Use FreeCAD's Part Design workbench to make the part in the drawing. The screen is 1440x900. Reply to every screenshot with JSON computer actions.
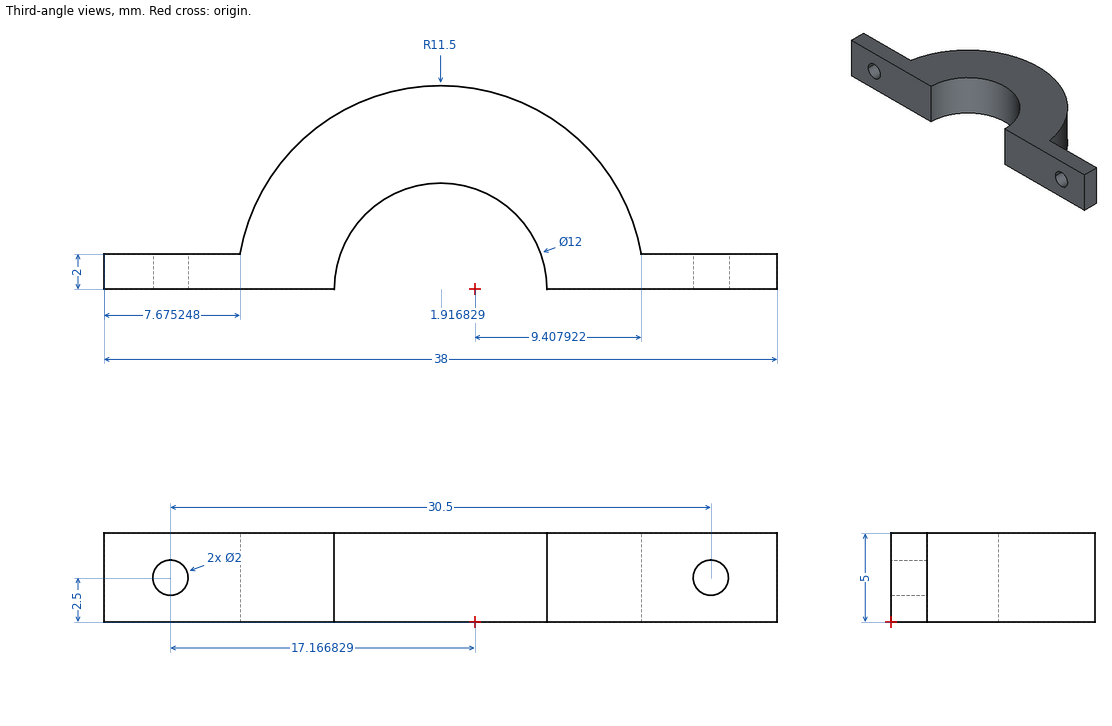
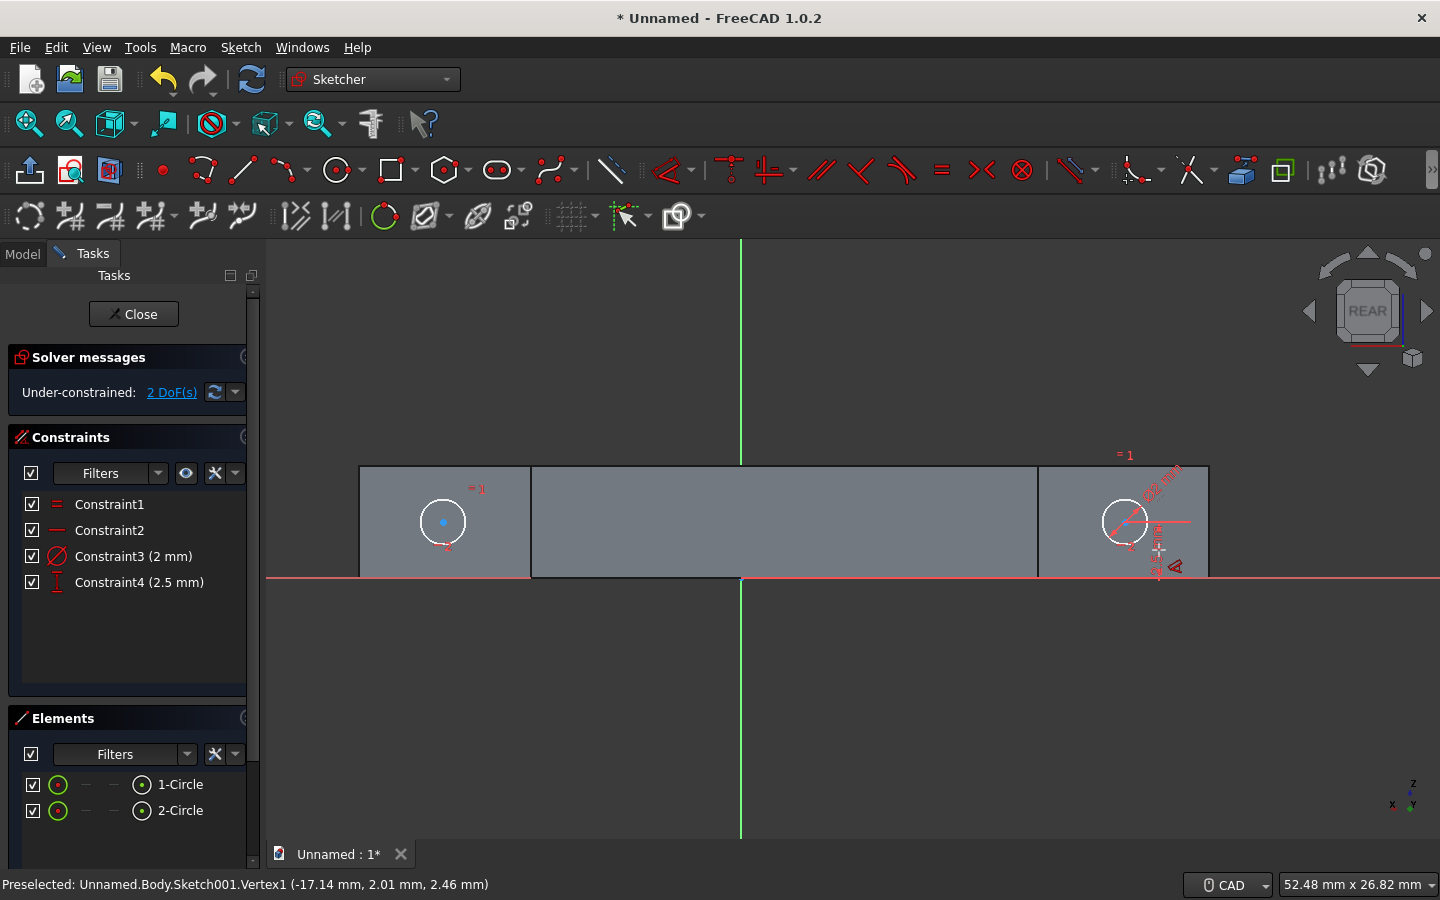
{"action": "left_click", "coordinate": [1125, 522]}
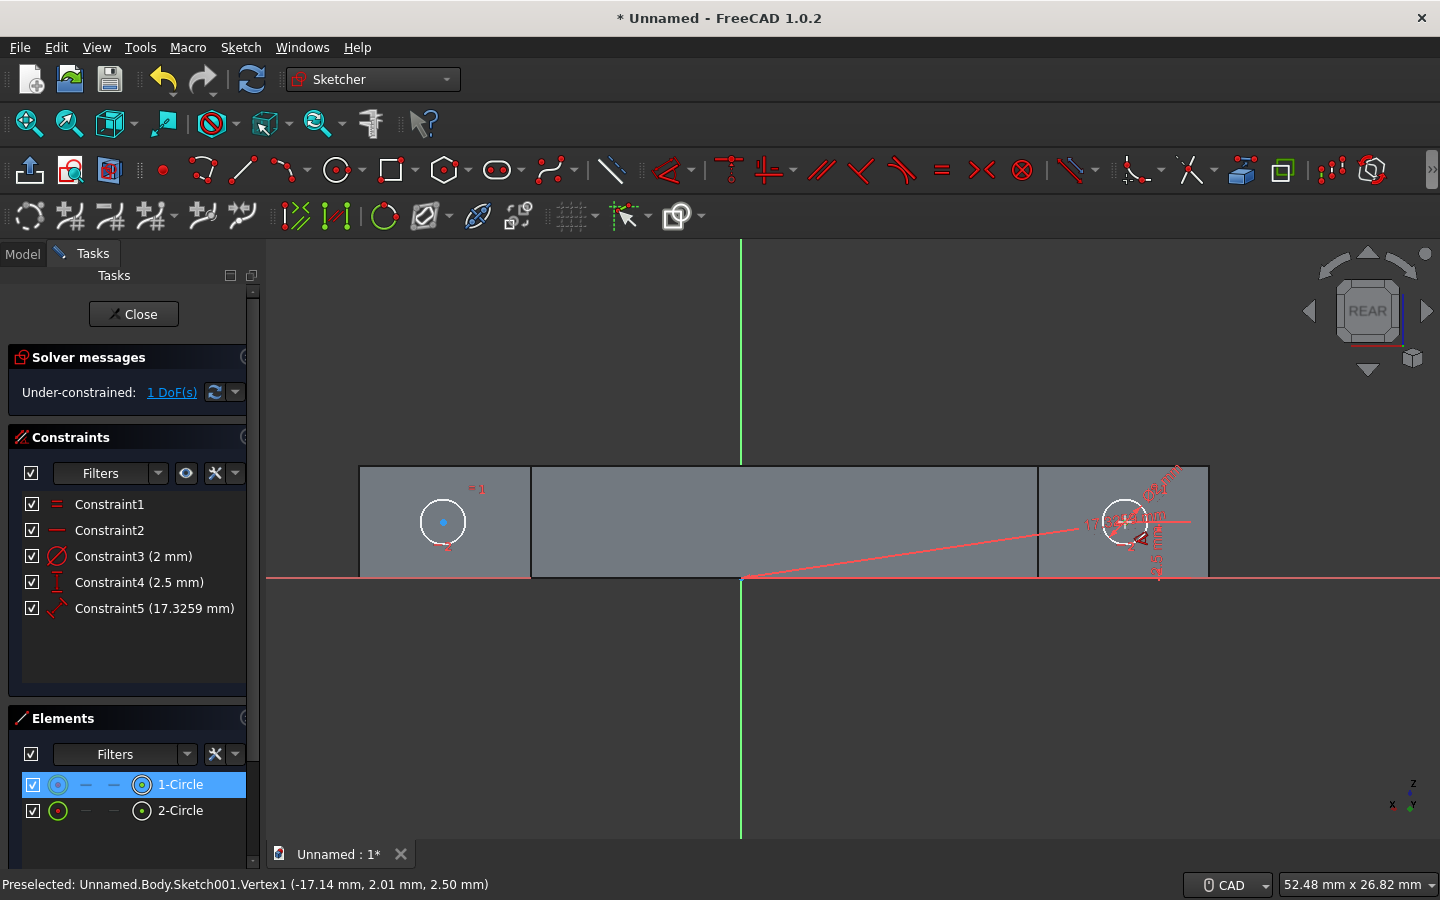
{"action": "left_click", "coordinate": [443, 522]}
{"action": "left_click", "coordinate": [784, 488]}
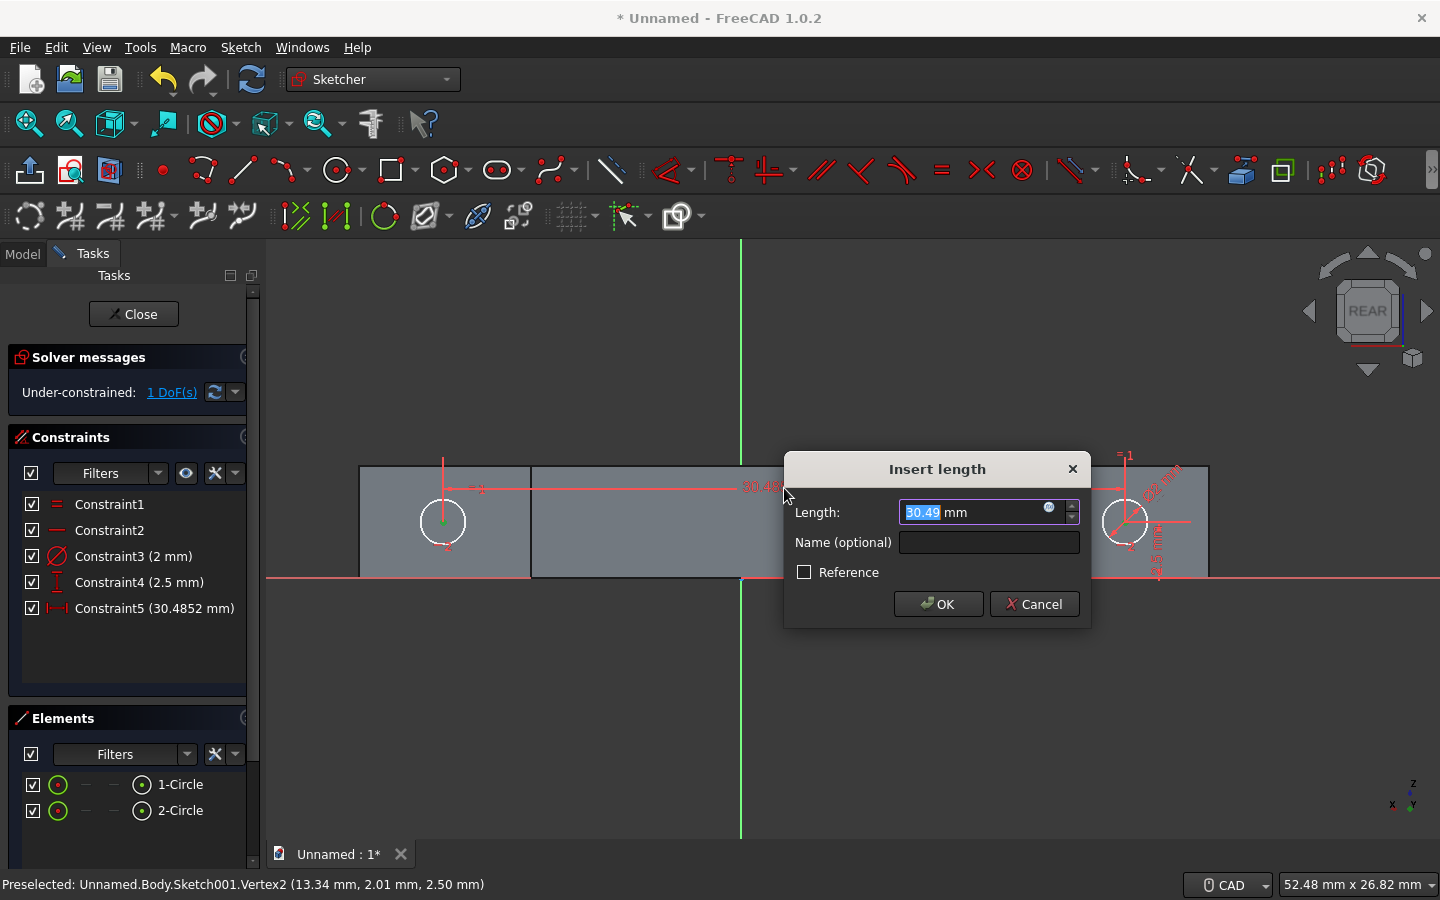
{"action": "type", "text": "30.5"}
{"action": "key", "text": "Return"}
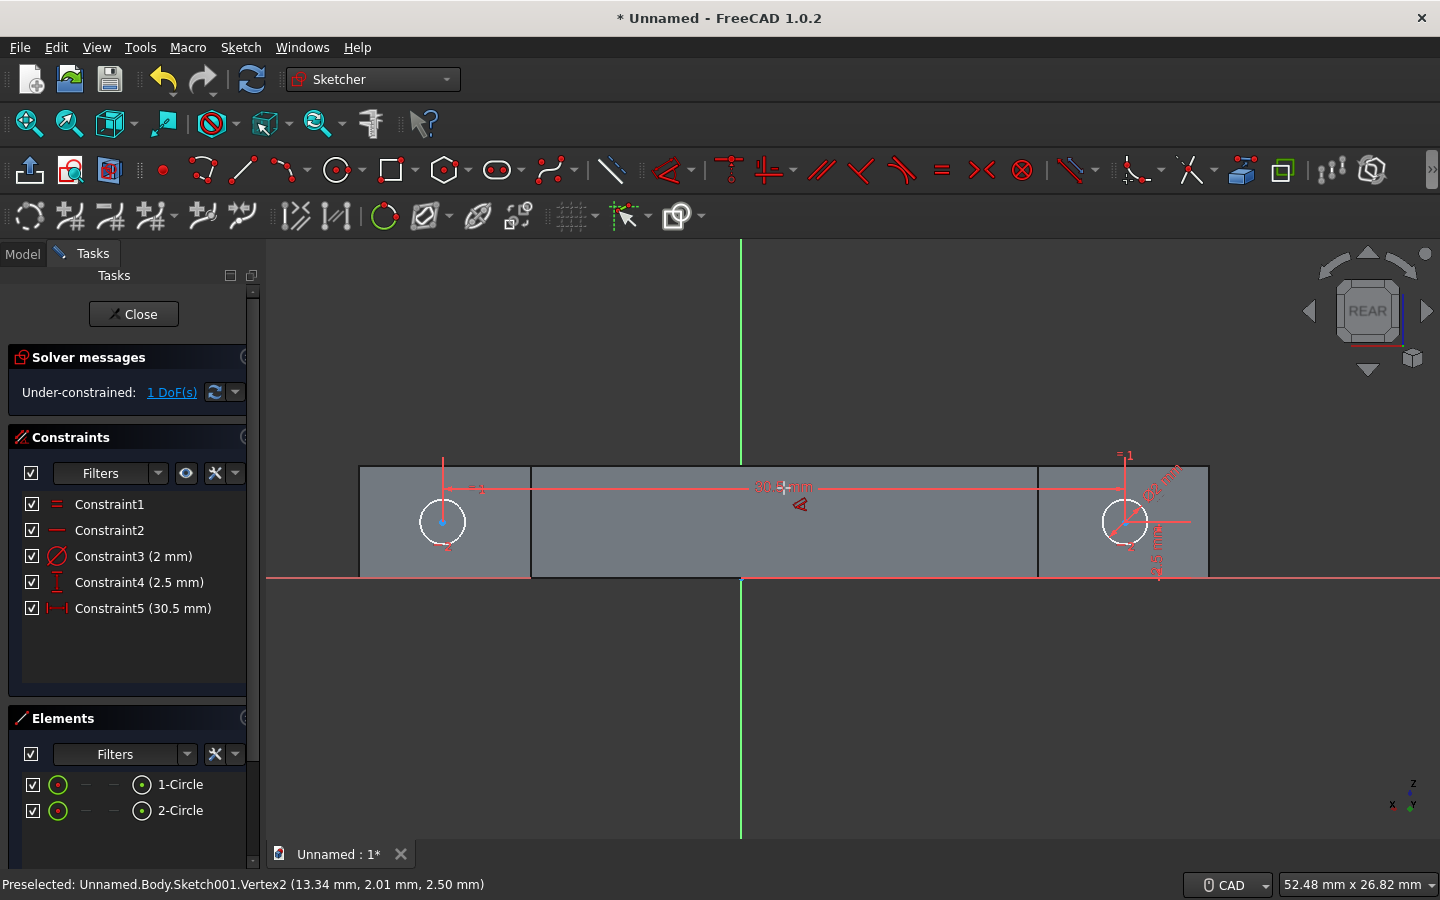
{"action": "left_click", "coordinate": [1125, 522]}
{"action": "left_click", "coordinate": [933, 612]}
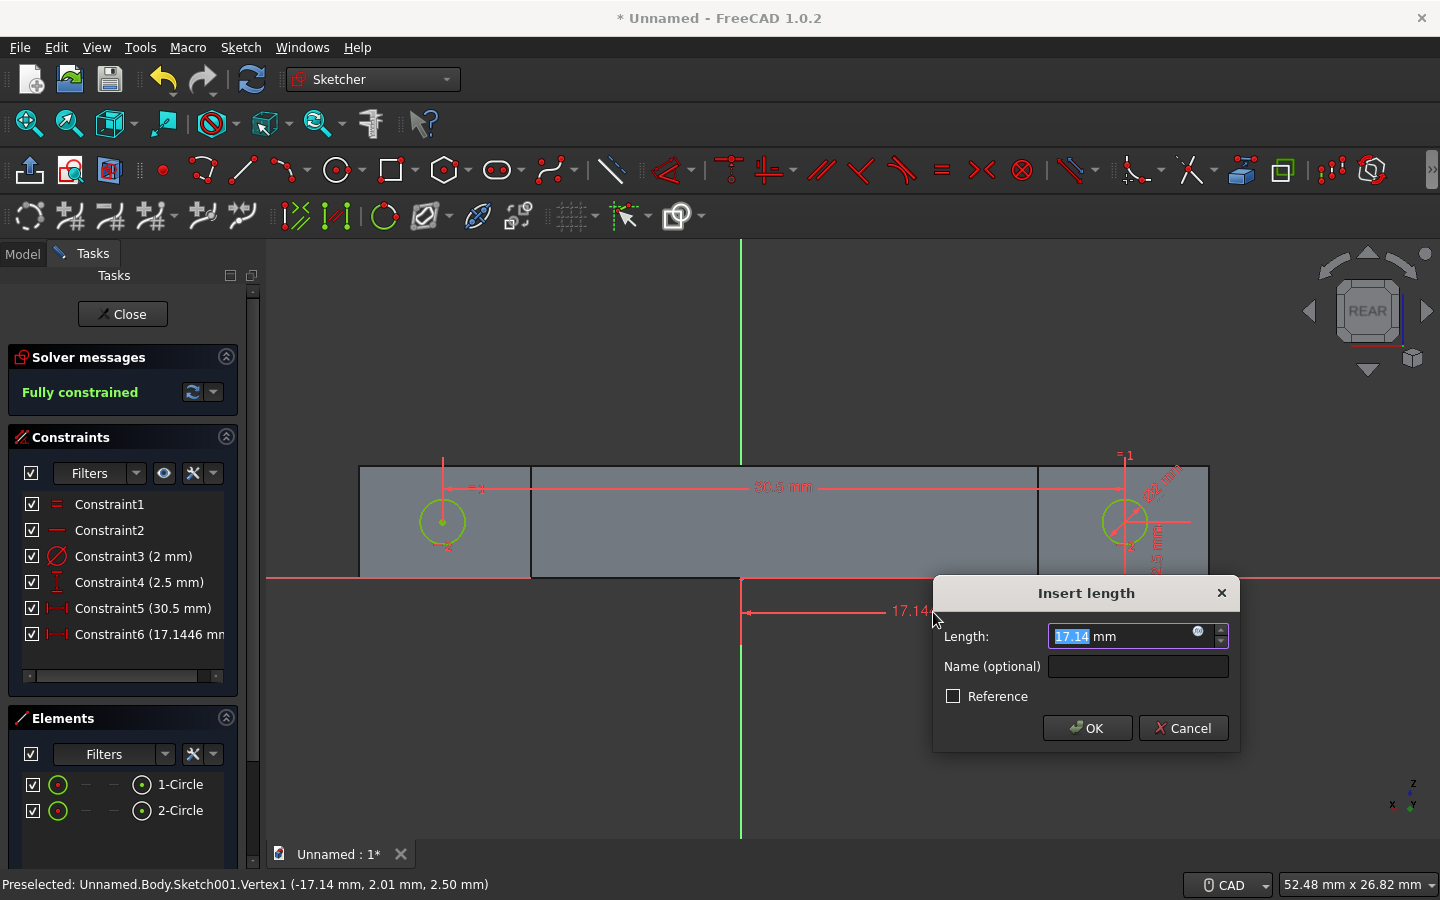
{"action": "type", "text": "17.166829"}
{"action": "key", "text": "Return"}
{"action": "key", "text": "Escape"}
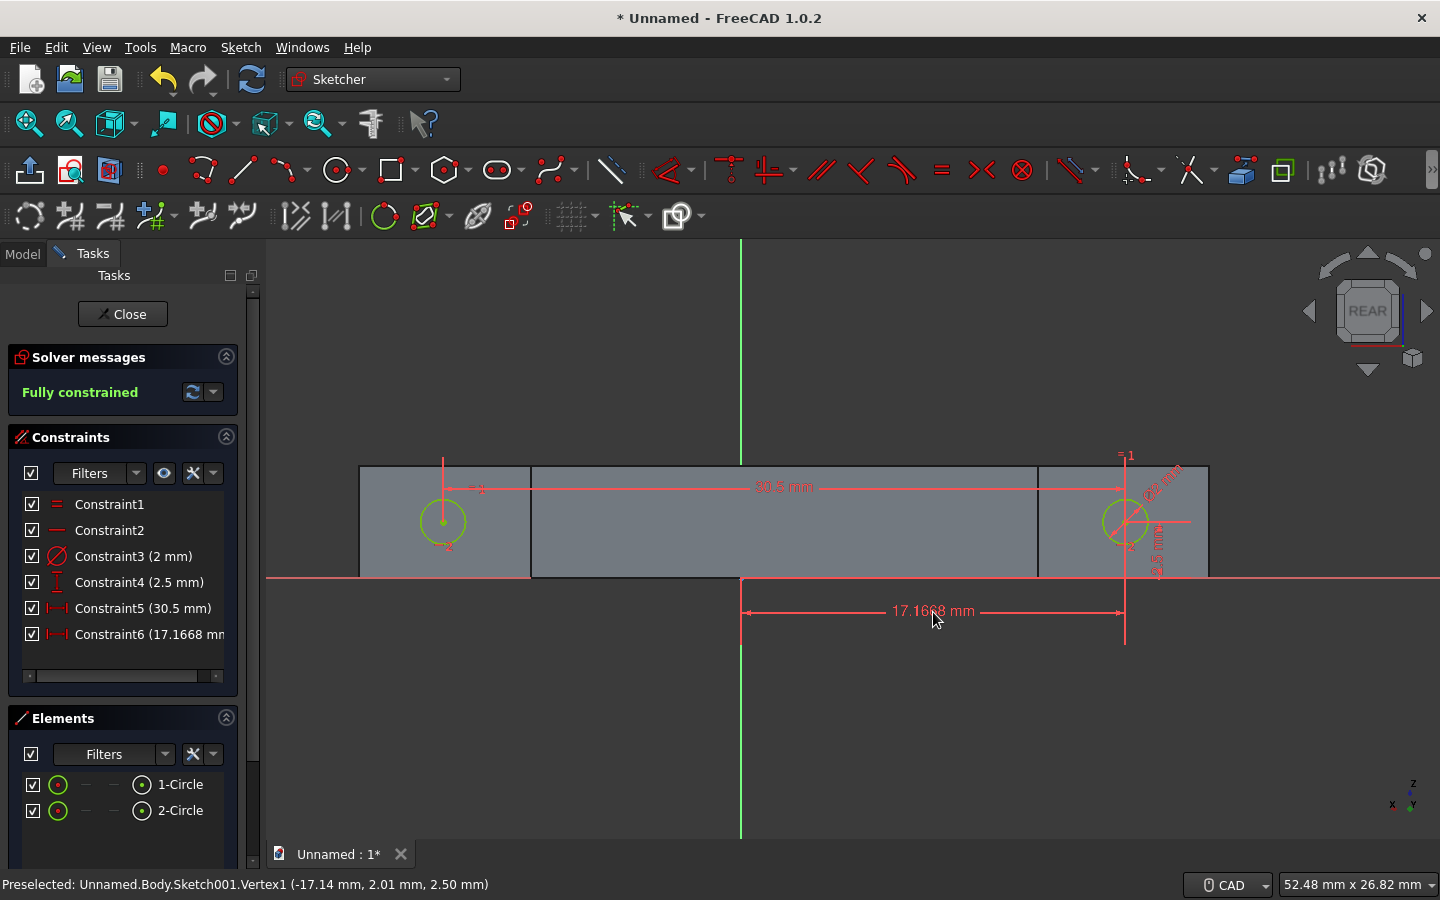
{"action": "left_click", "coordinate": [123, 314]}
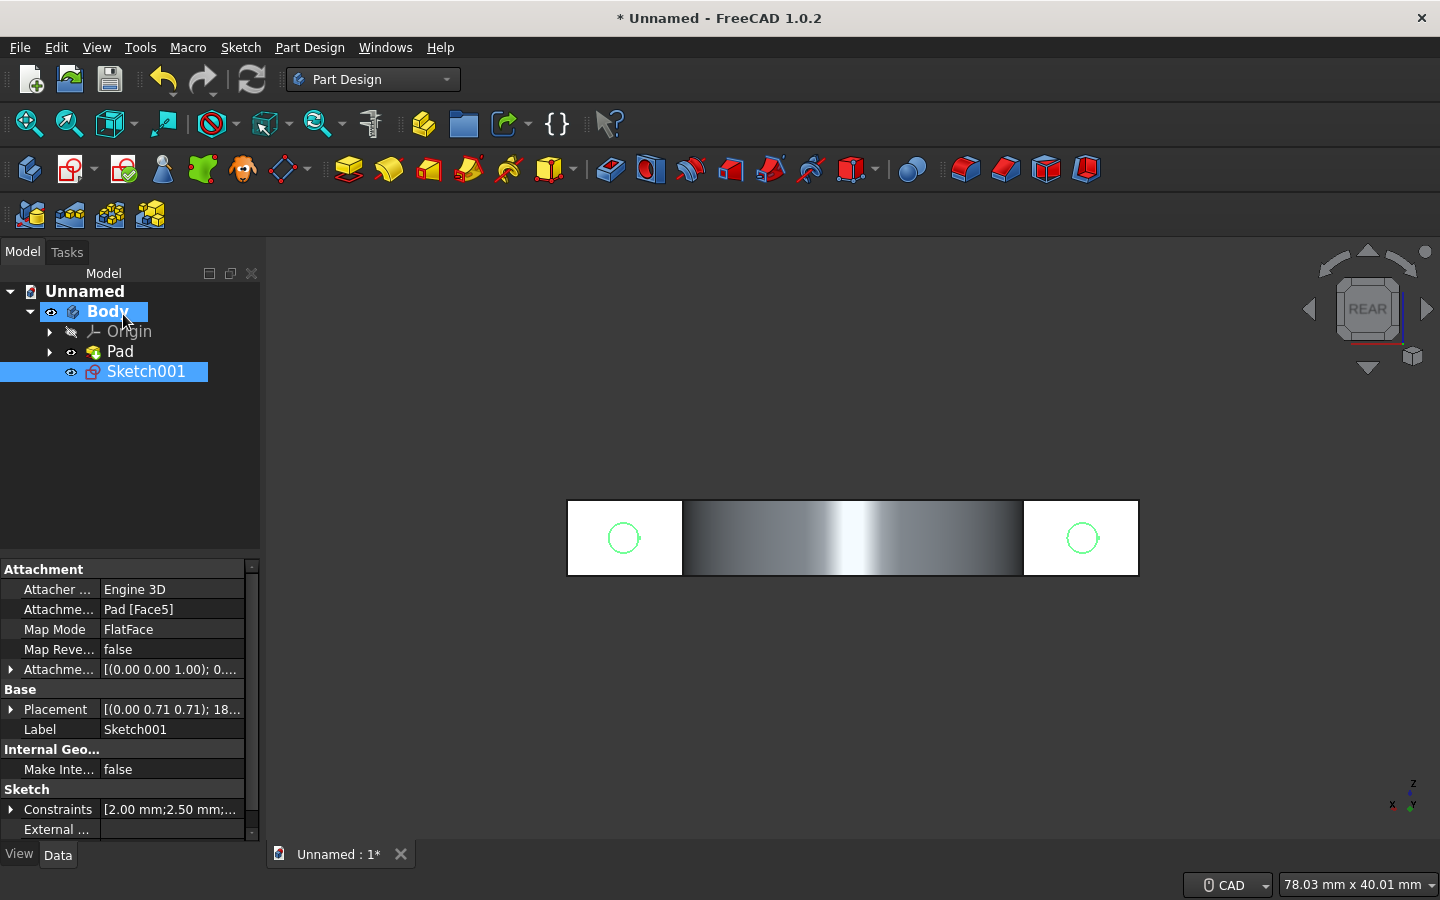
{"action": "left_click", "coordinate": [612, 170]}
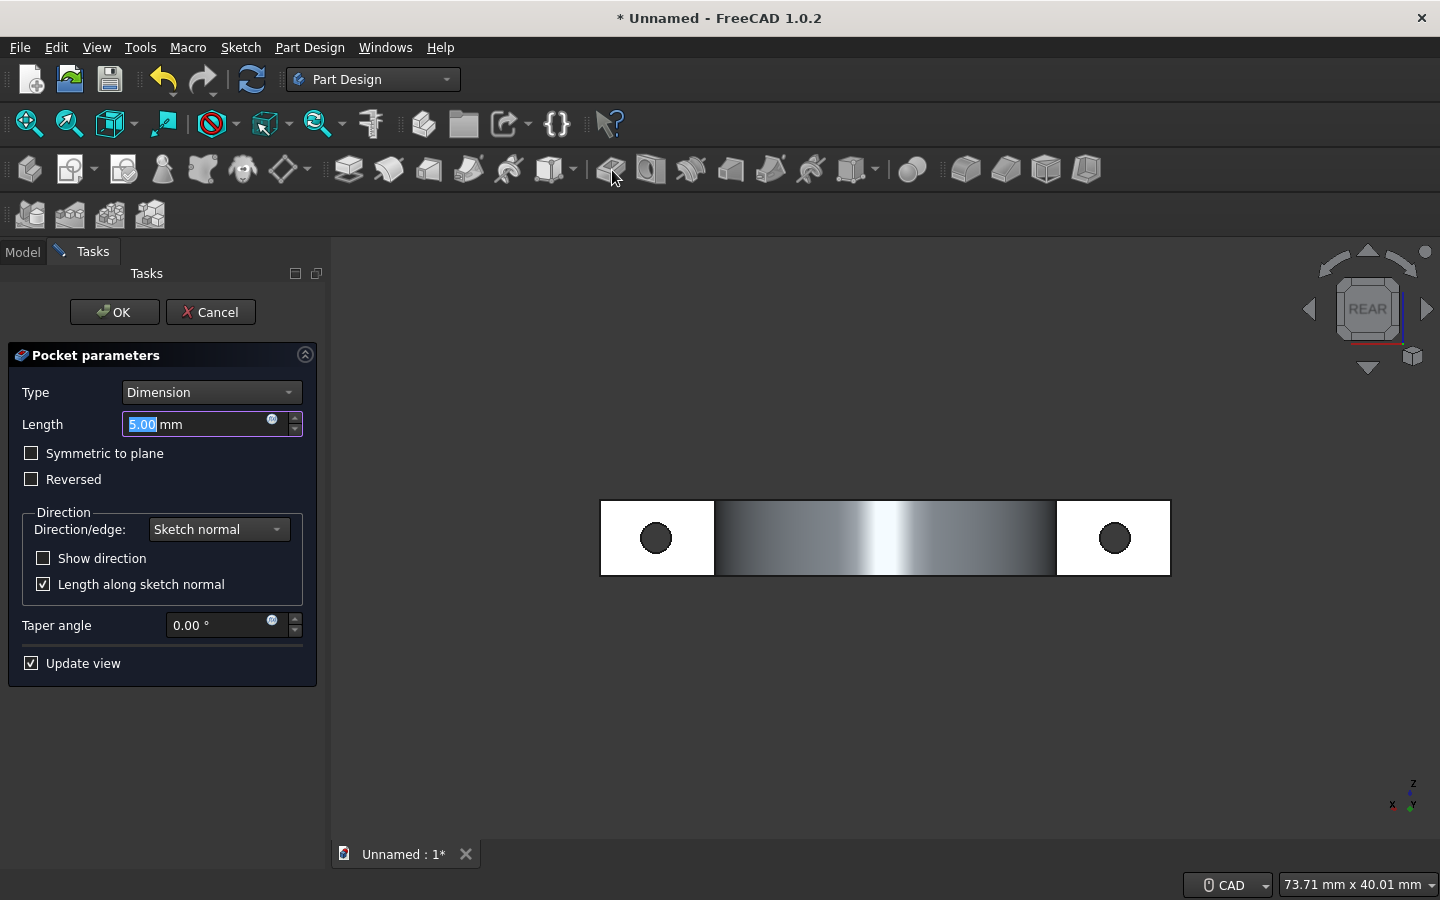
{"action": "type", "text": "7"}
{"action": "key", "text": "Tab"}